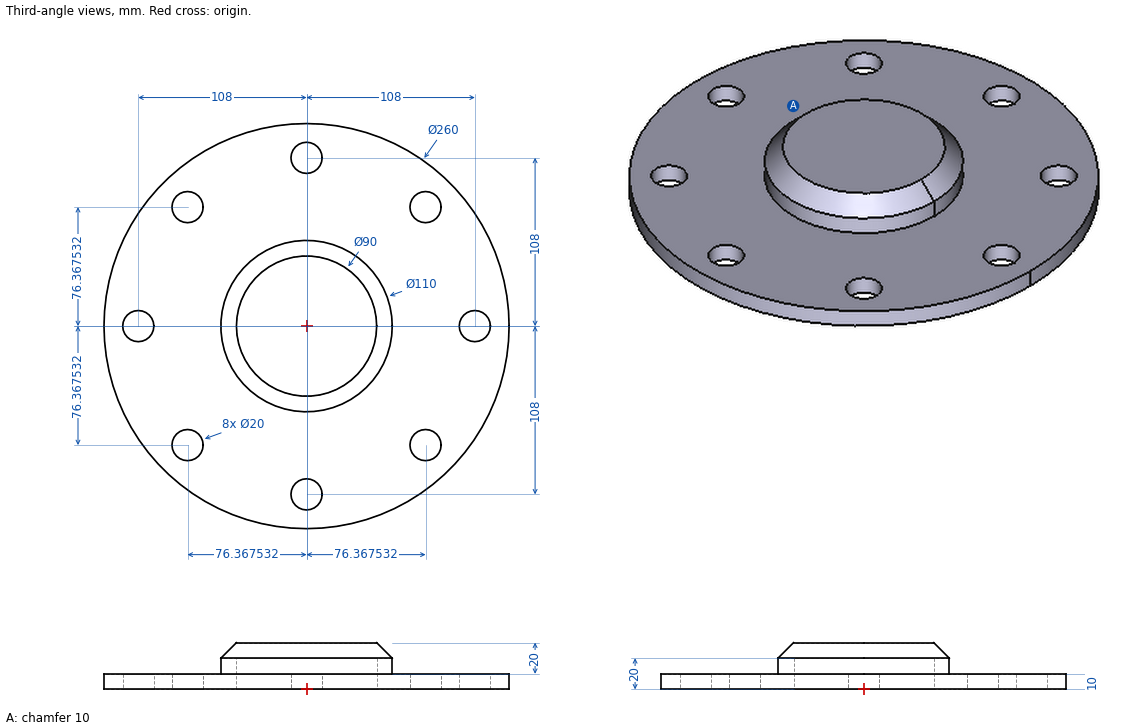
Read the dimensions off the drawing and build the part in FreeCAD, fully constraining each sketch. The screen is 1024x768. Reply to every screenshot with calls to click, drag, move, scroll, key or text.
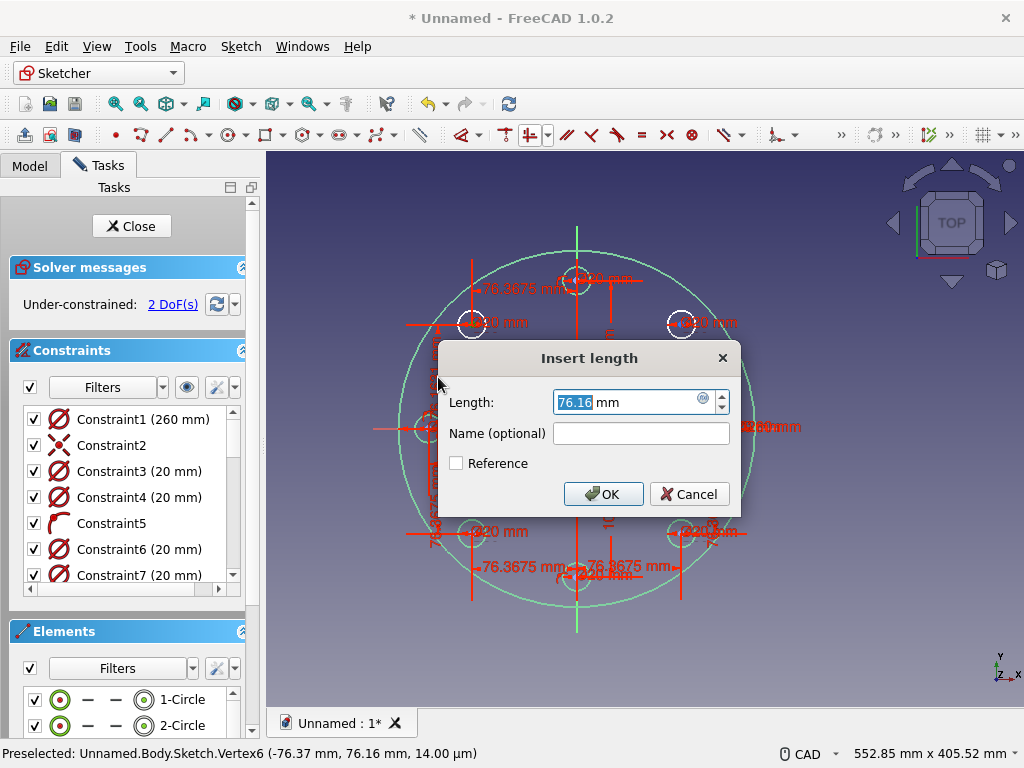
text(76.367532)
key(Return)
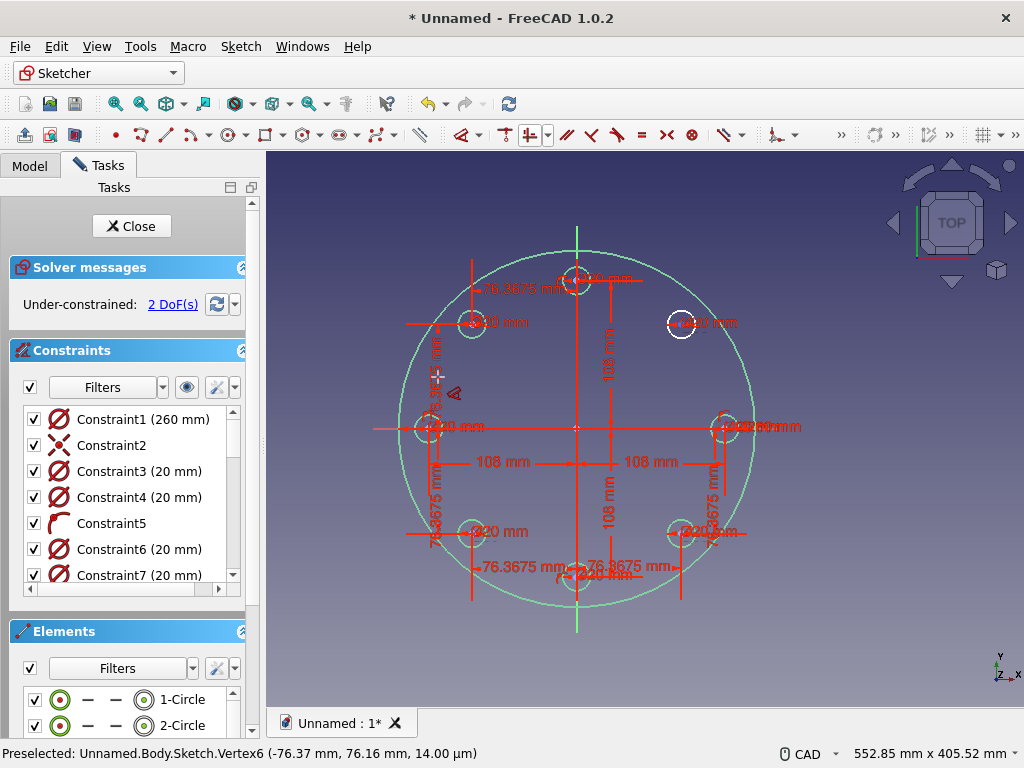
click(681, 325)
click(629, 291)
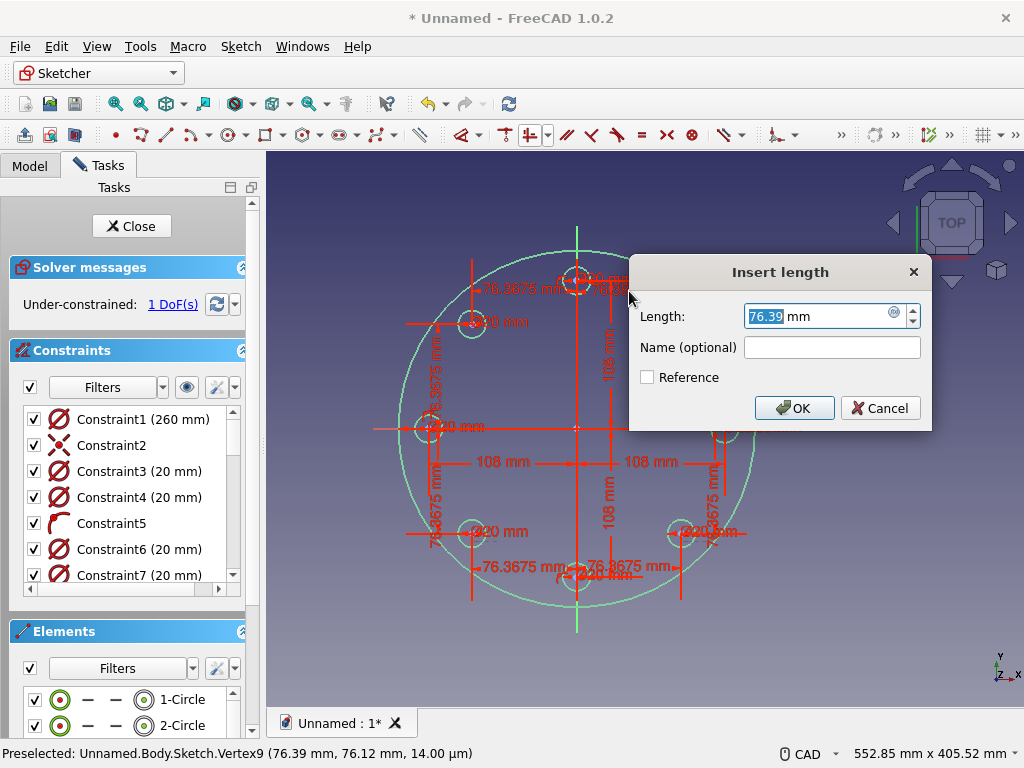
text(76.367532)
key(Return)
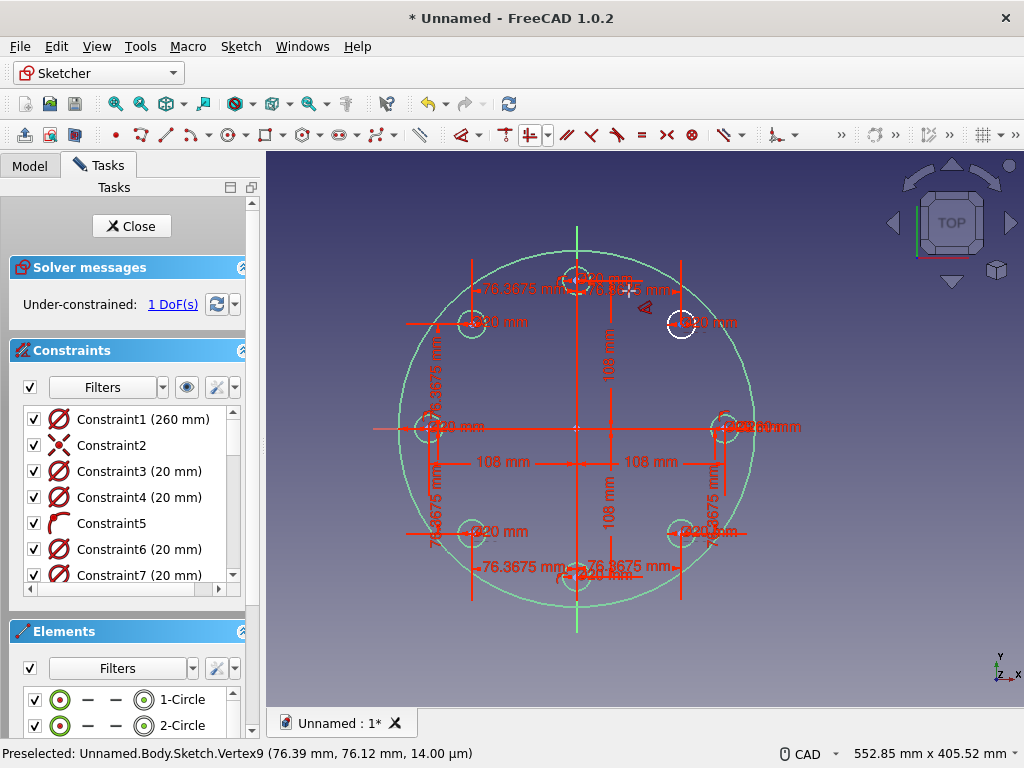
click(681, 325)
click(715, 377)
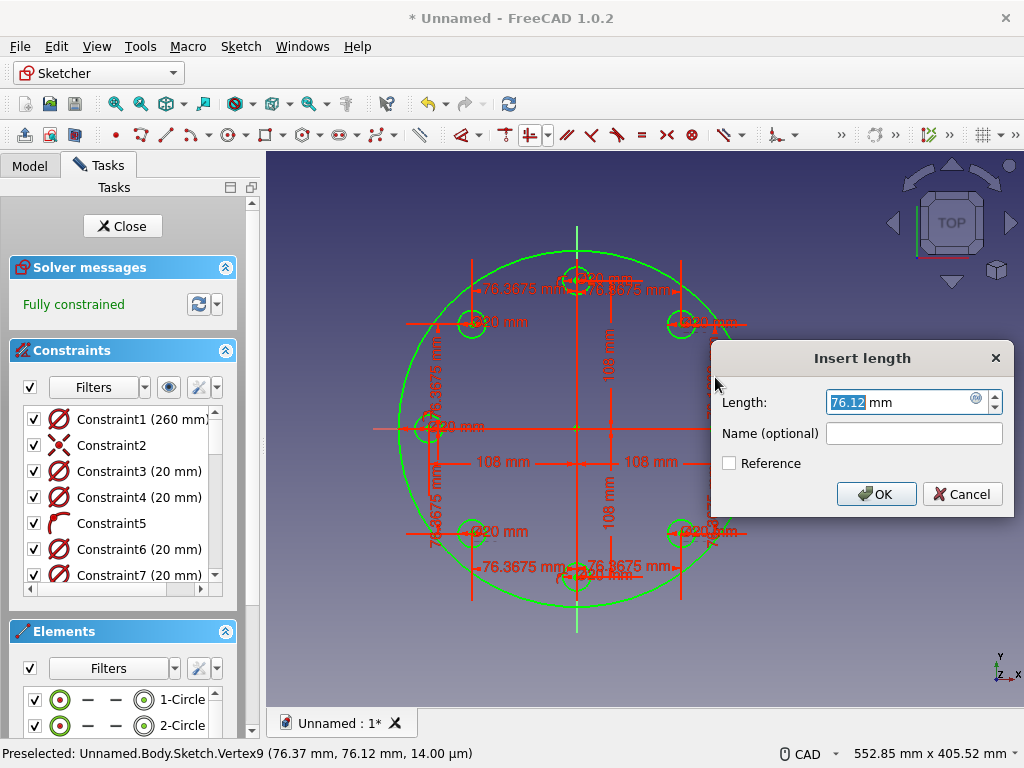
text(76.367532)
key(Return)
key(Escape)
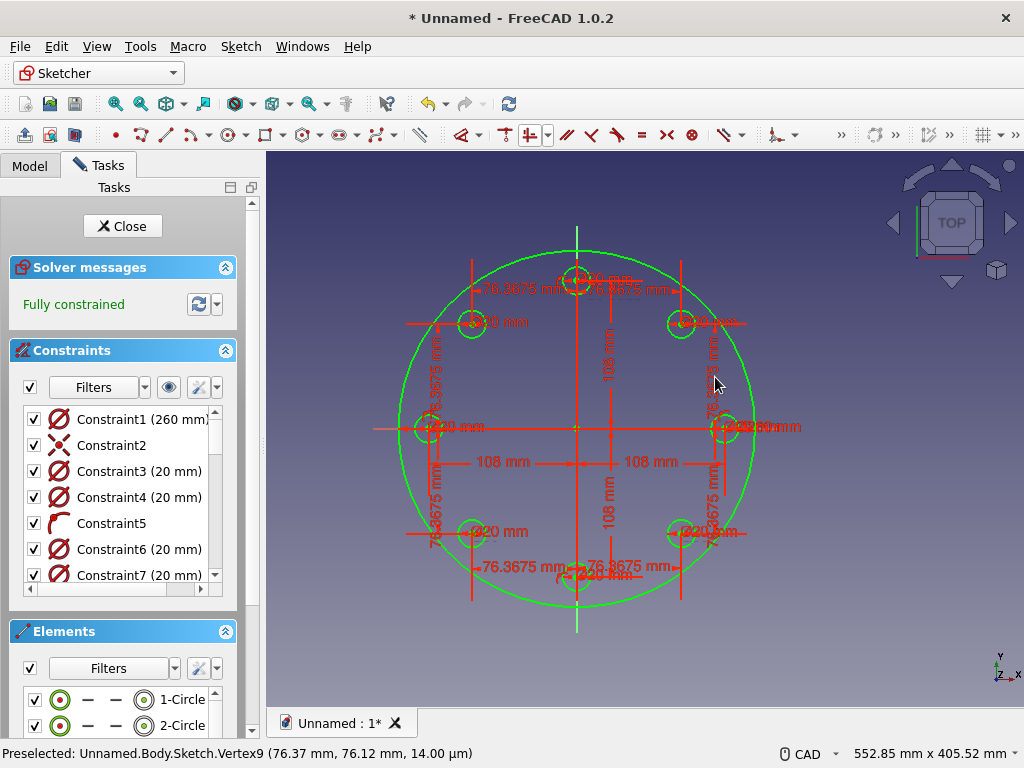
click(123, 226)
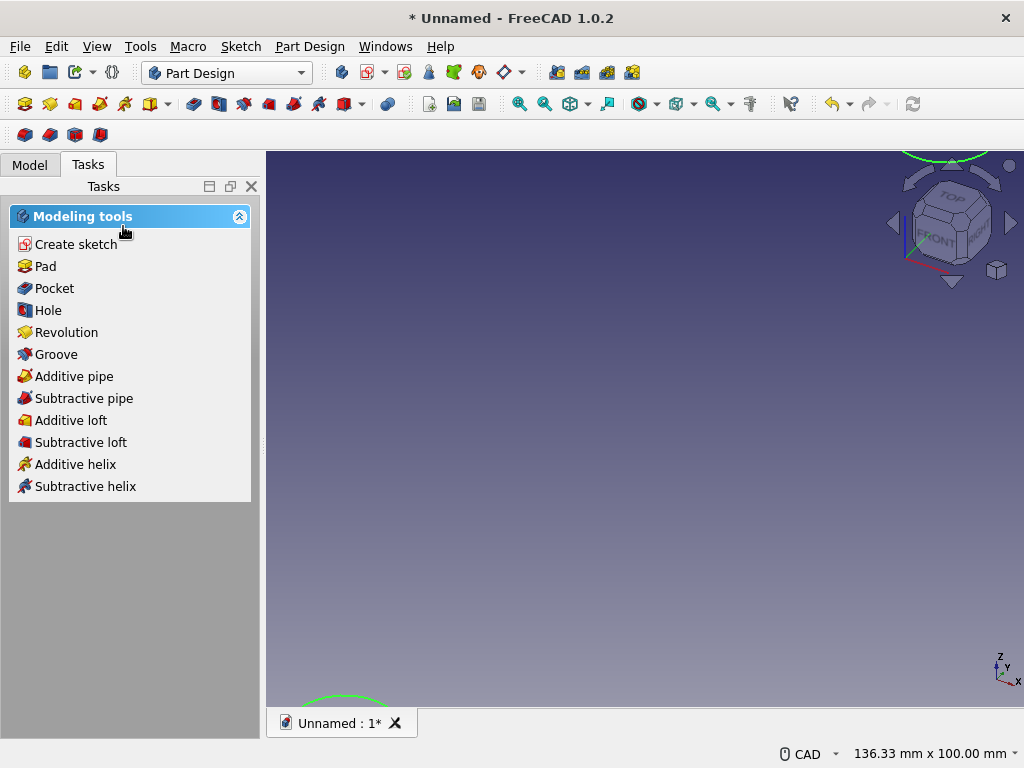
click(25, 104)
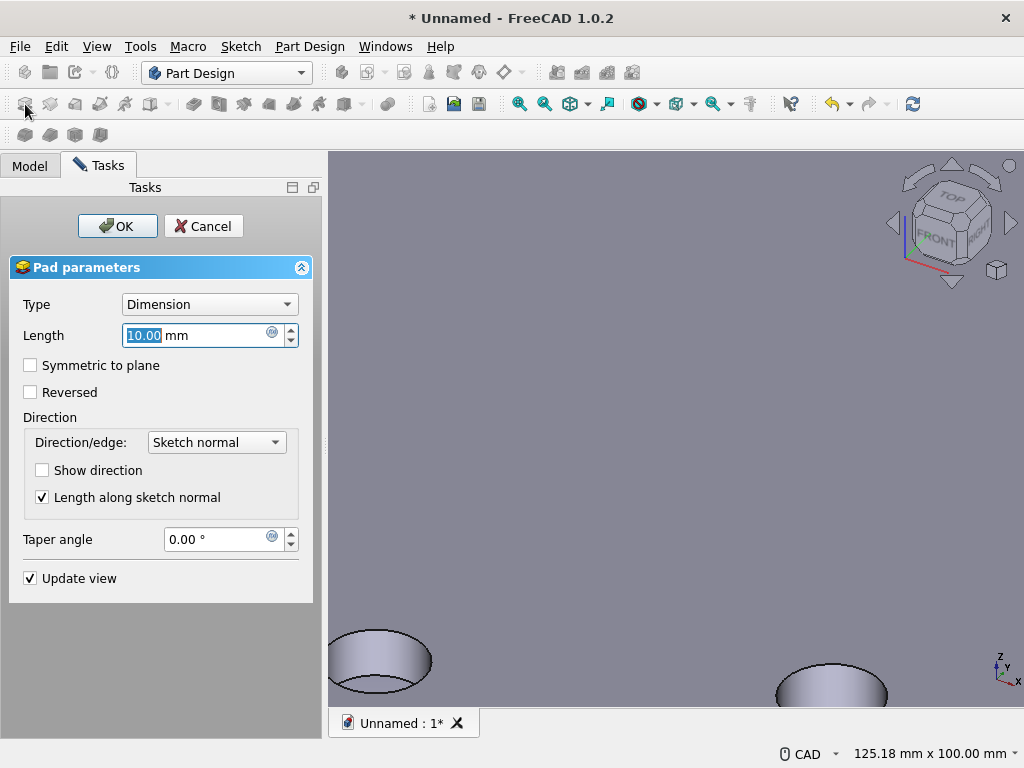
text(10)
key(Tab)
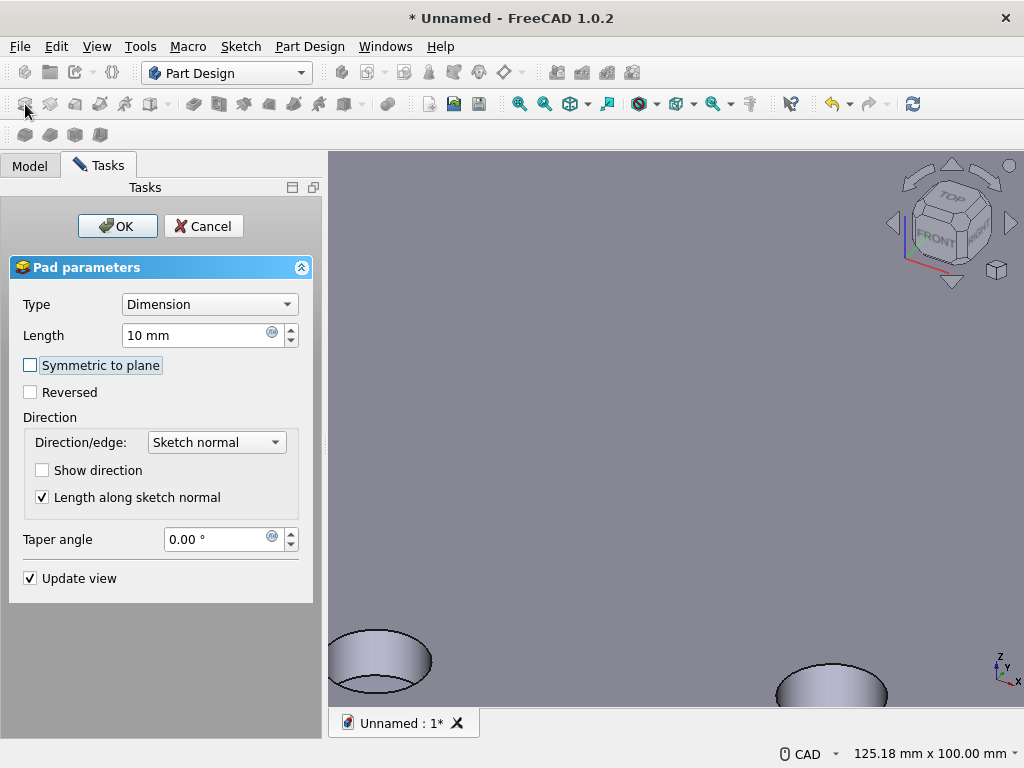
click(118, 226)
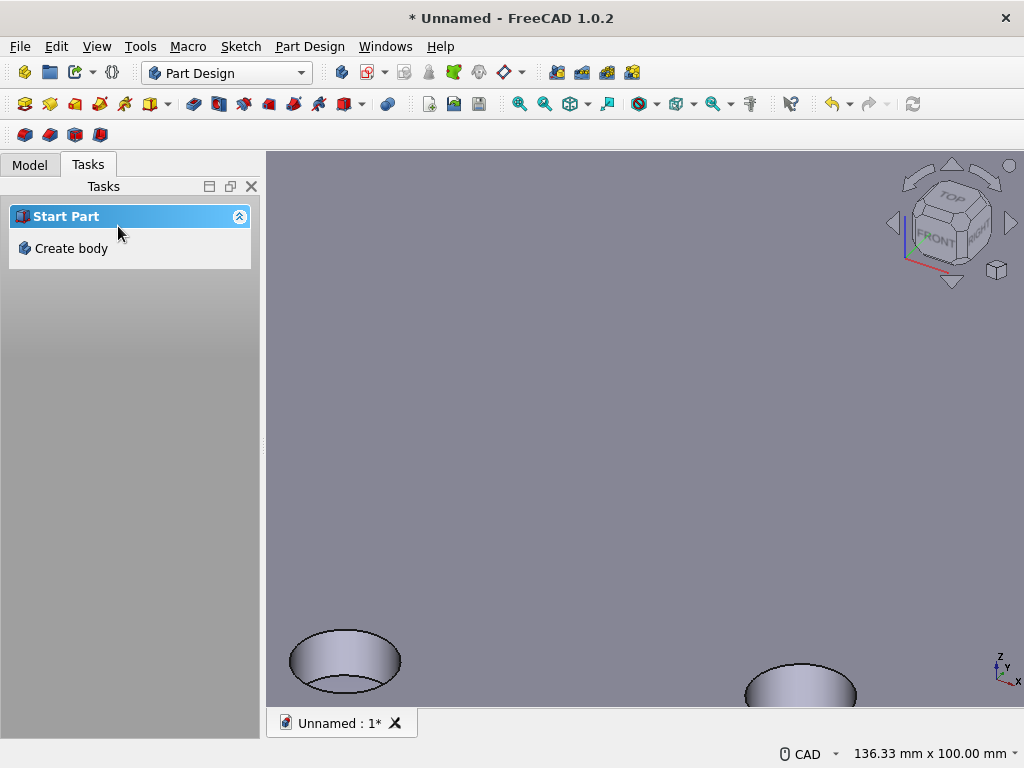
key(v)
key(f)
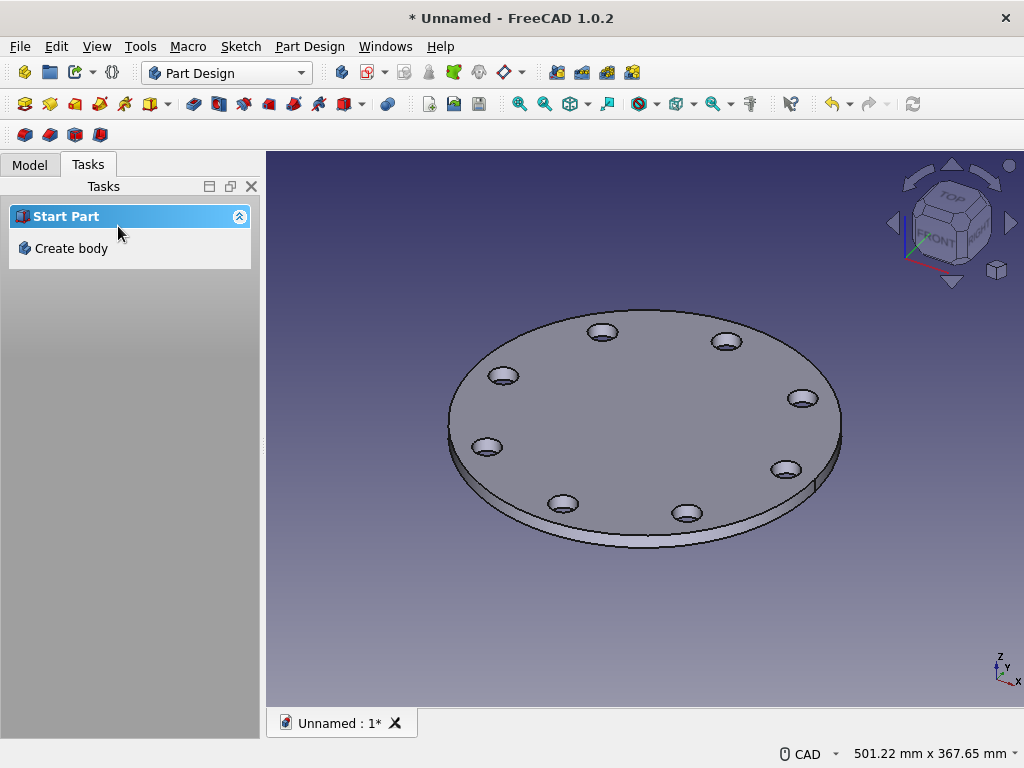
click(645, 422)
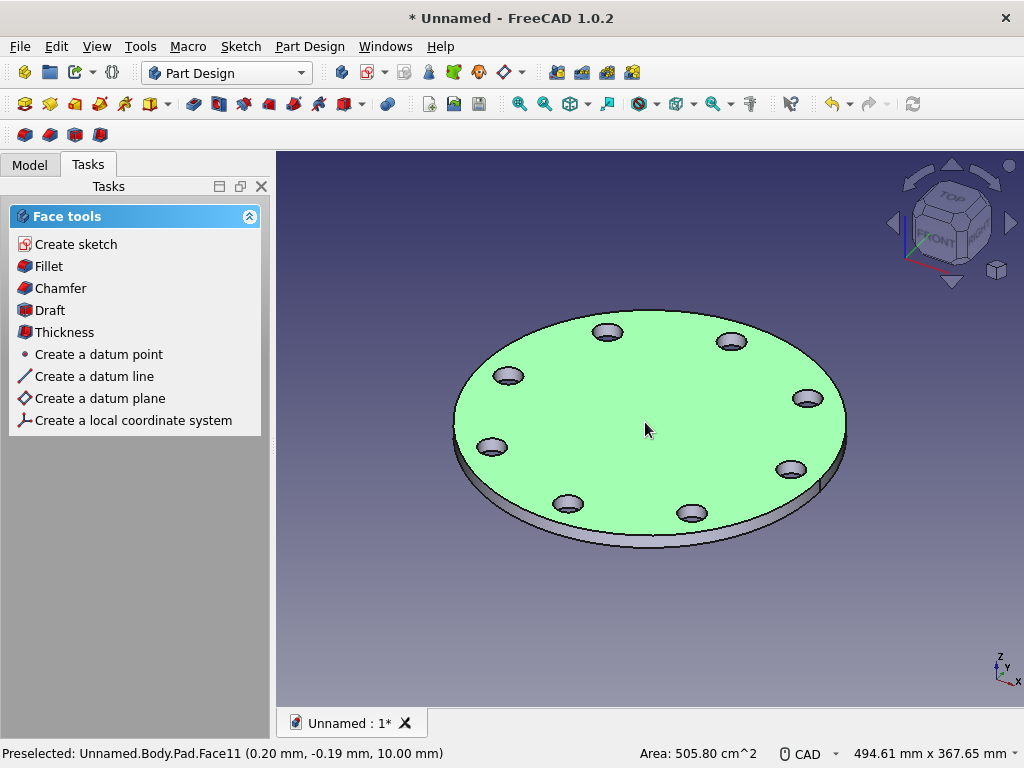
click(366, 72)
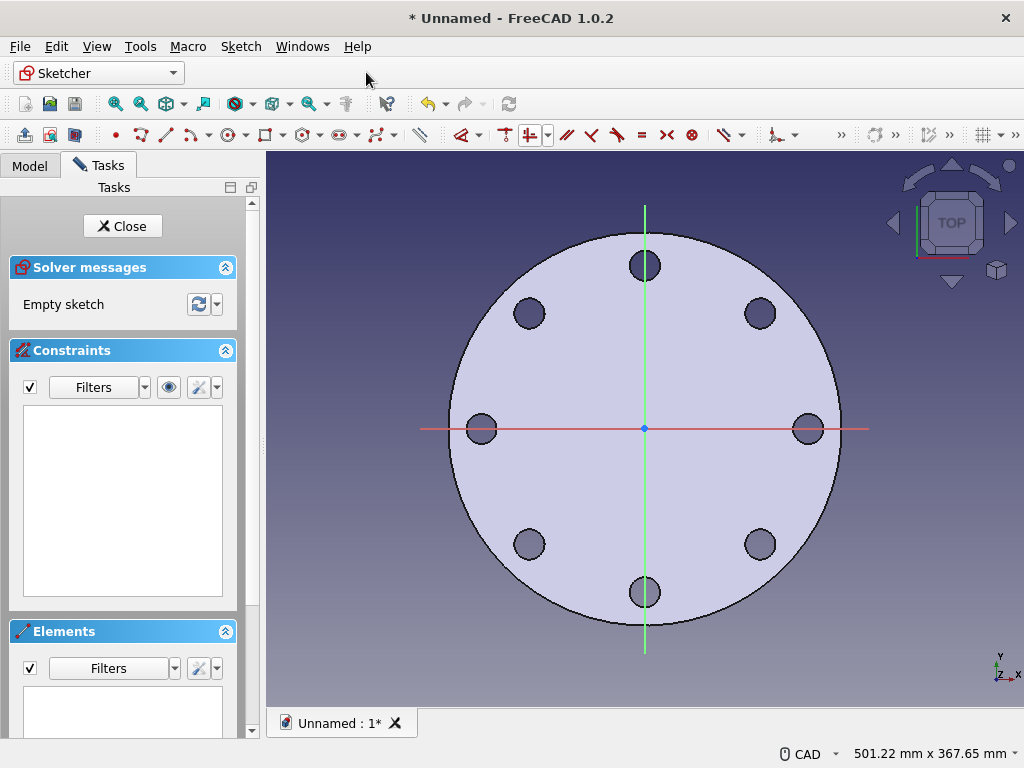
scroll(701, 429, up, 4)